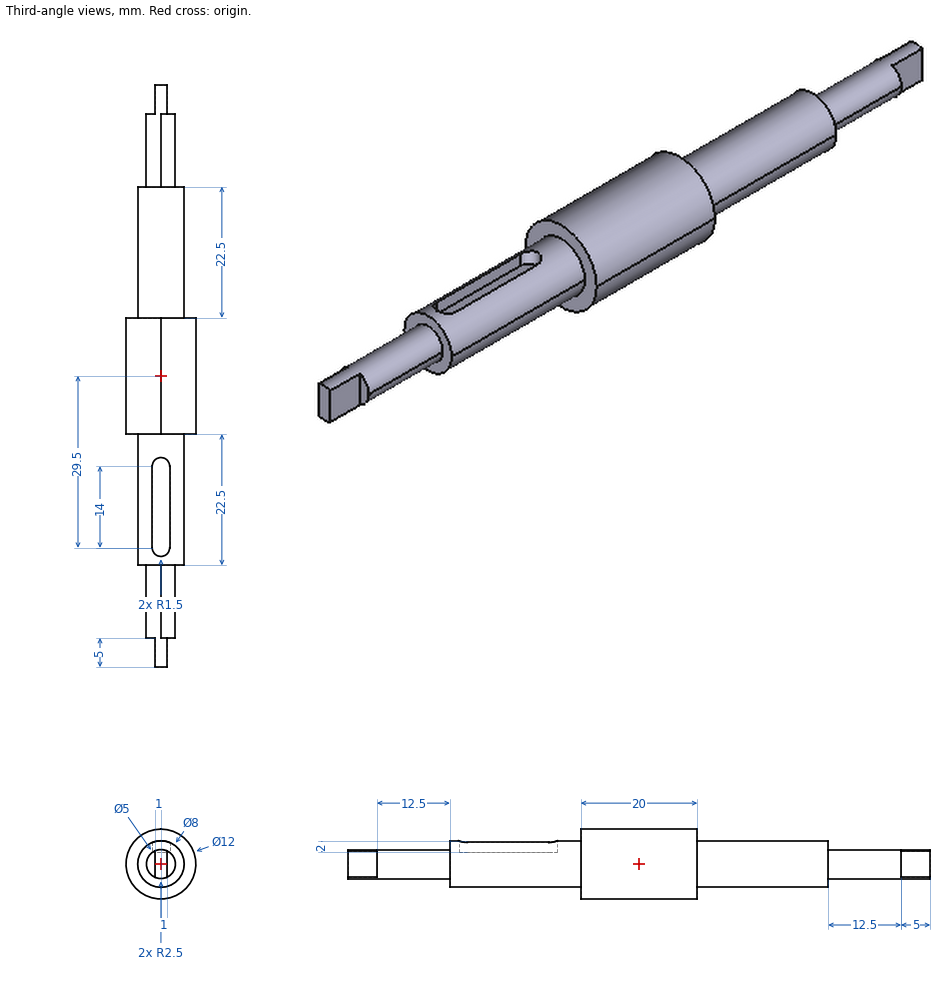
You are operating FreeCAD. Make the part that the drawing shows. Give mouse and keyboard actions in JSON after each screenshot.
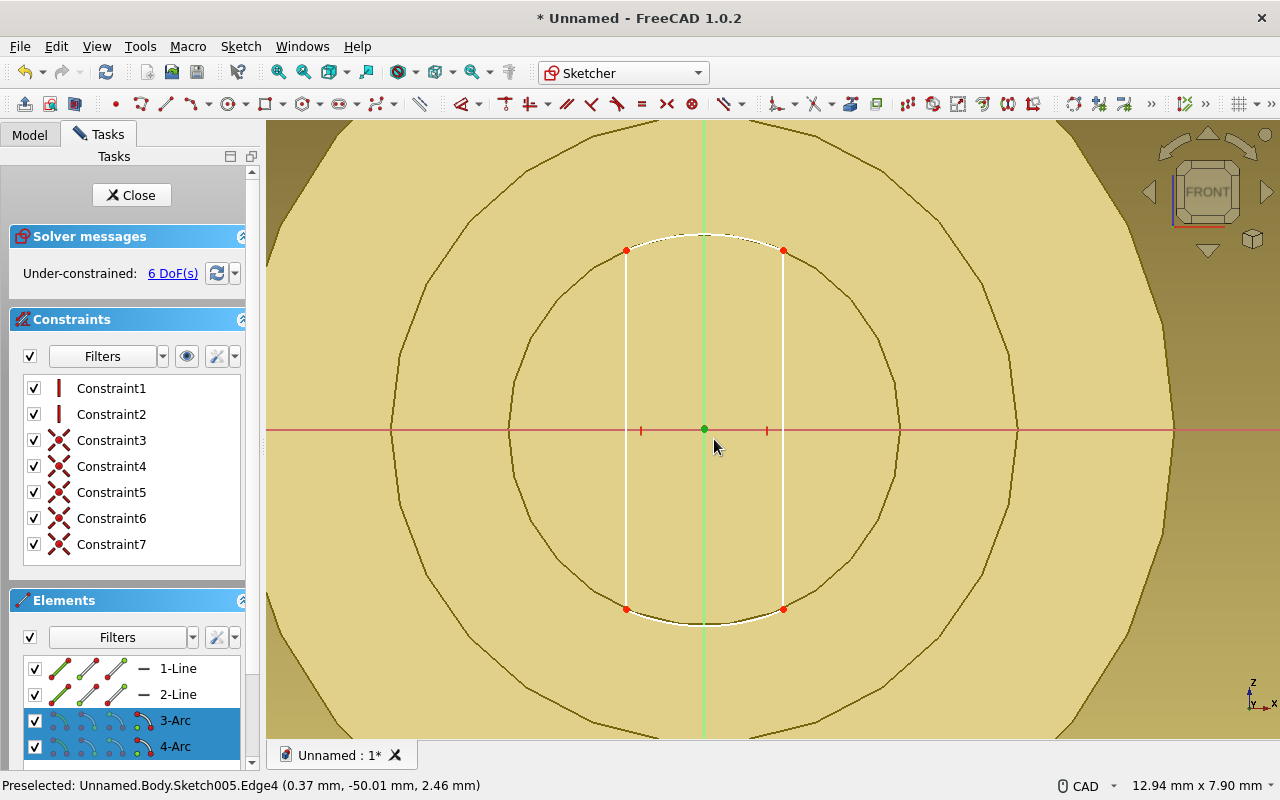
{"action": "left_click", "coordinate": [505, 104]}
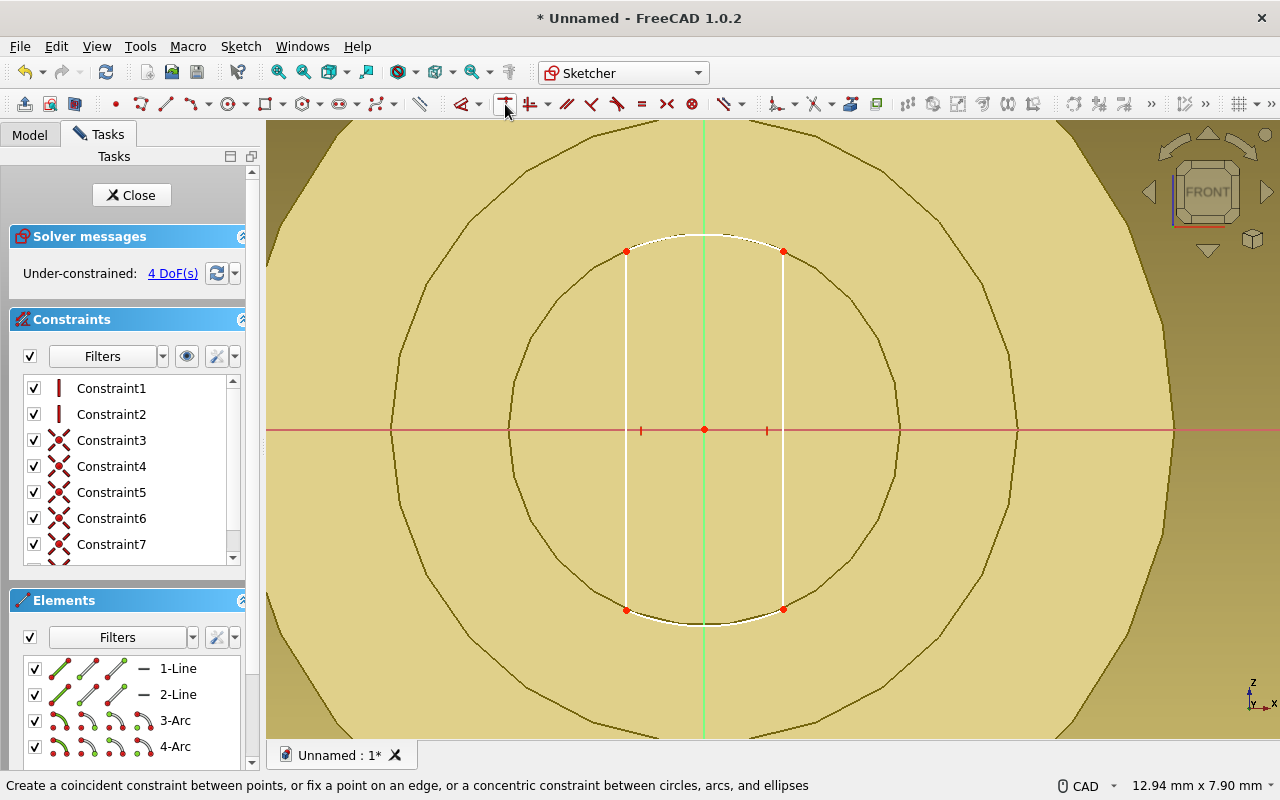
{"action": "left_click", "coordinate": [672, 624]}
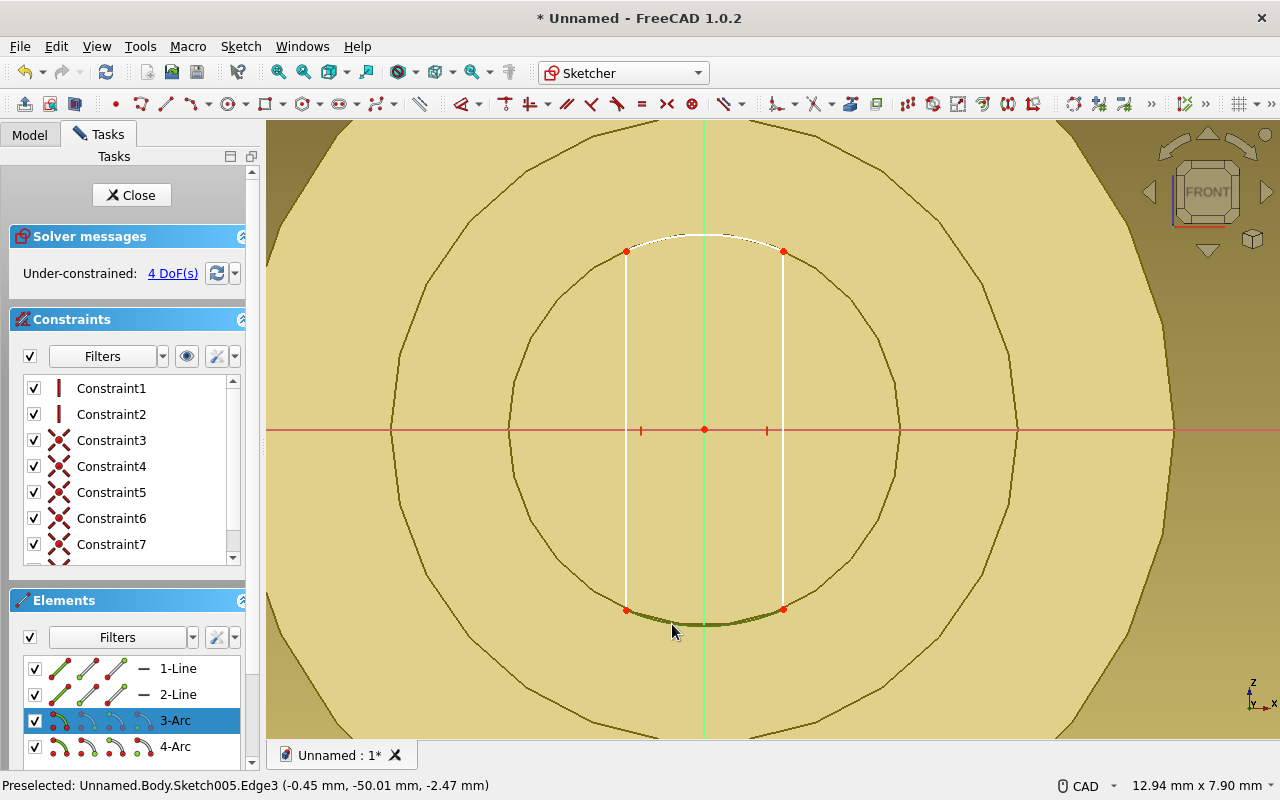
{"action": "left_click", "coordinate": [737, 237]}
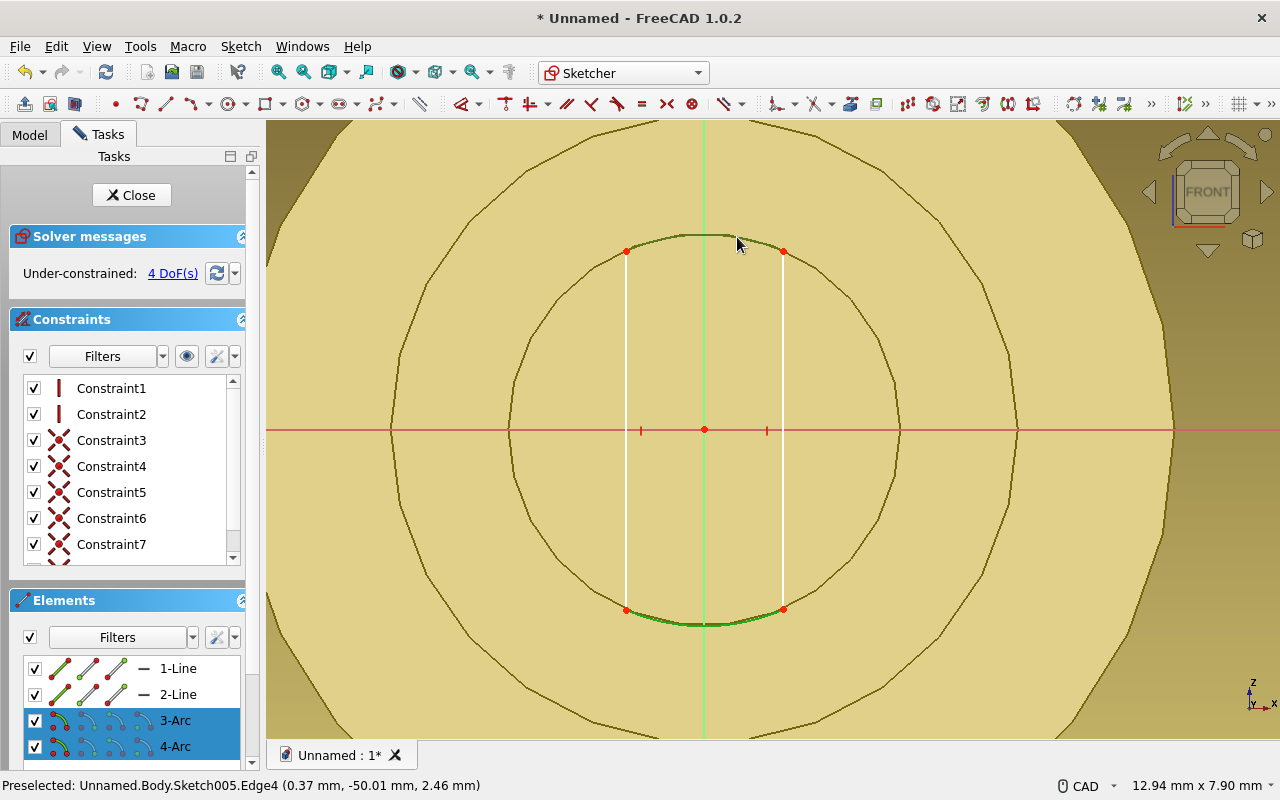
{"action": "key", "text": "e"}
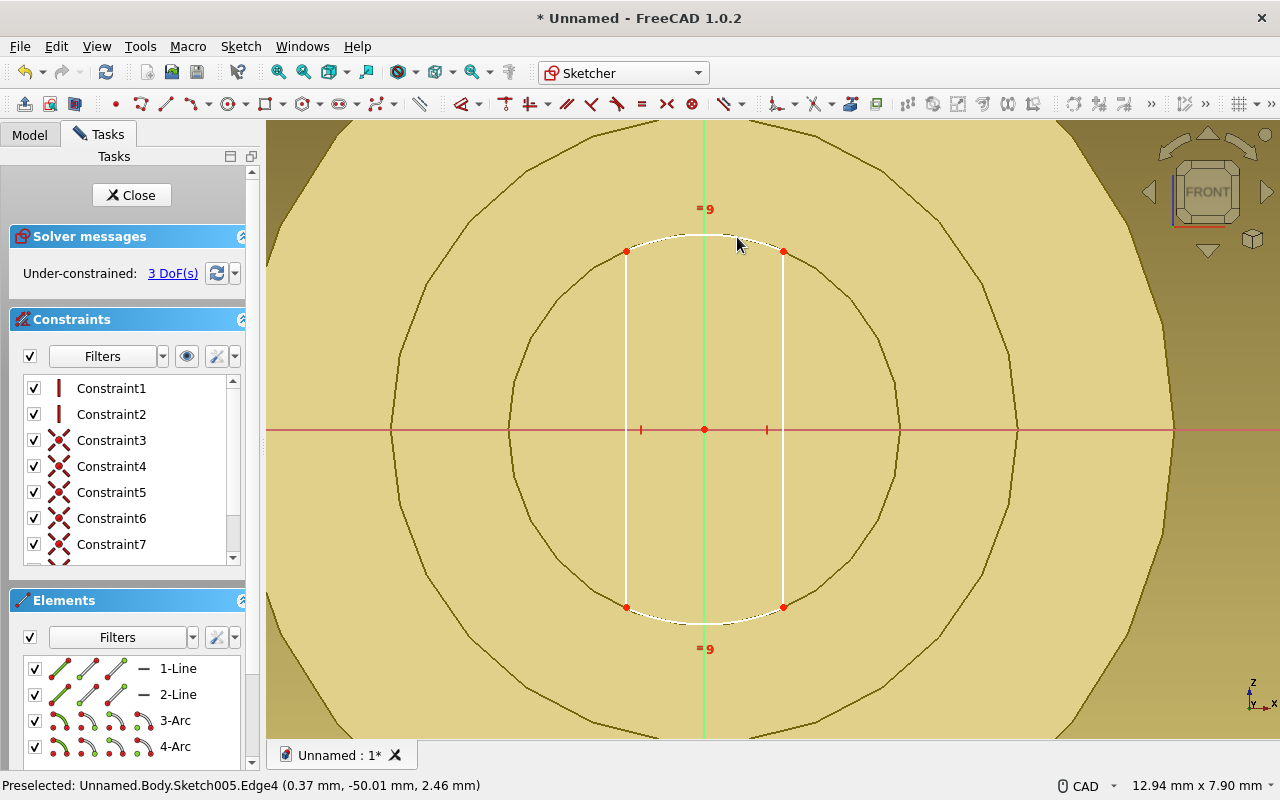
{"action": "key", "text": "d"}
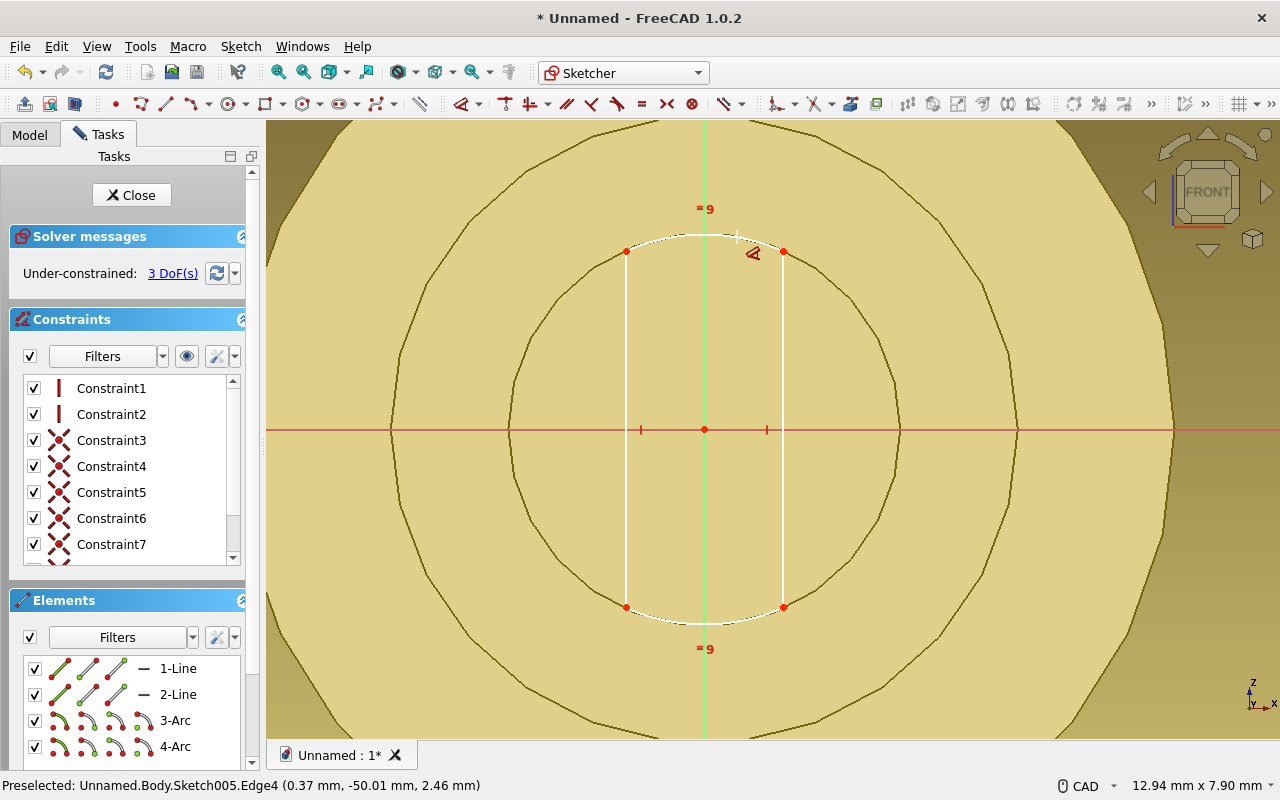
{"action": "left_click", "coordinate": [672, 622]}
{"action": "left_click", "coordinate": [667, 654]}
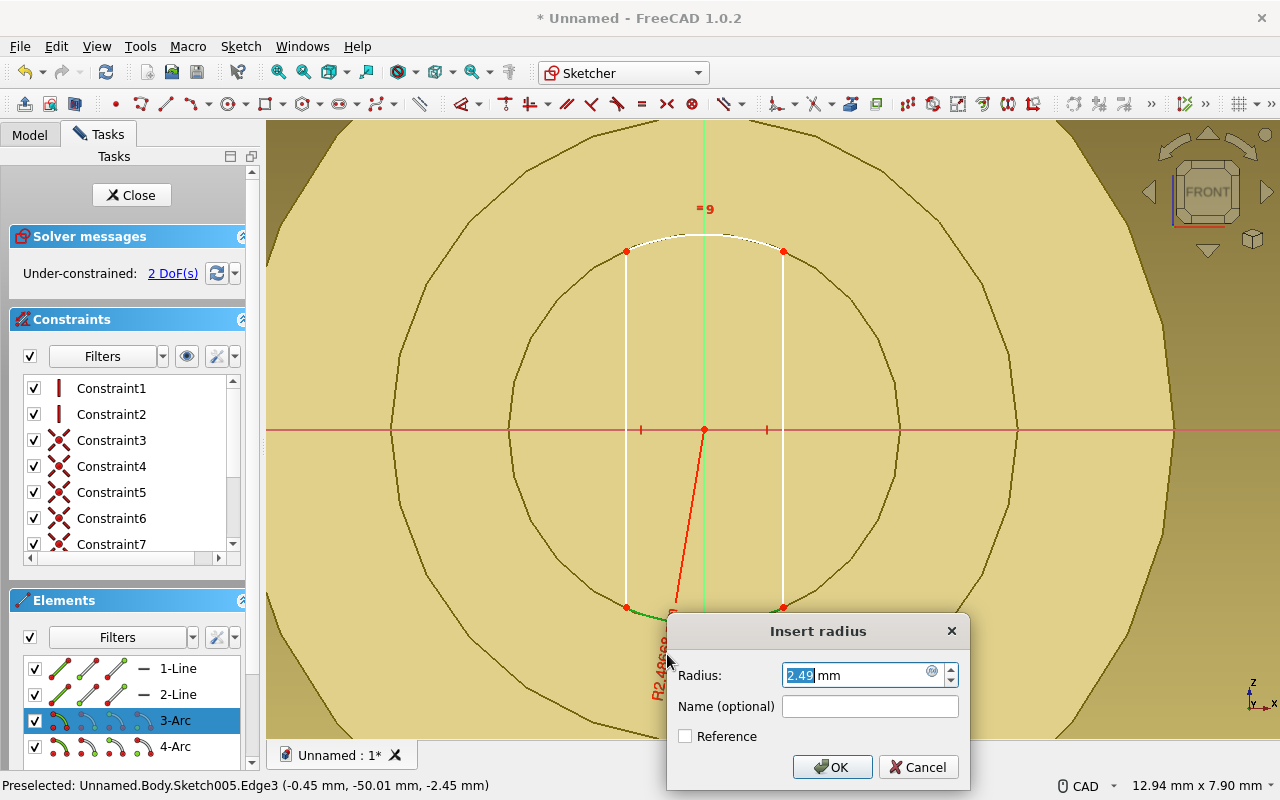
{"action": "type", "text": "2.5"}
{"action": "key", "text": "Return"}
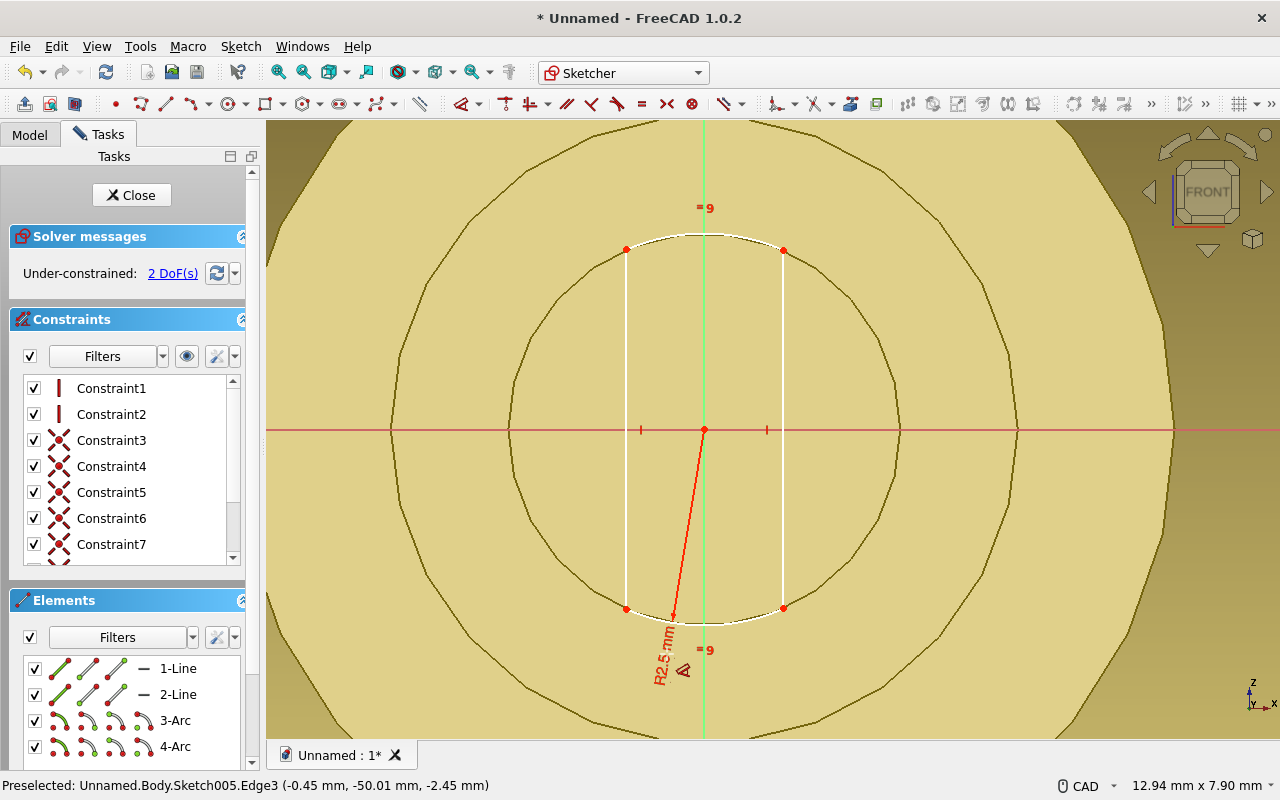
{"action": "left_click", "coordinate": [626, 250]}
{"action": "left_click", "coordinate": [665, 216]}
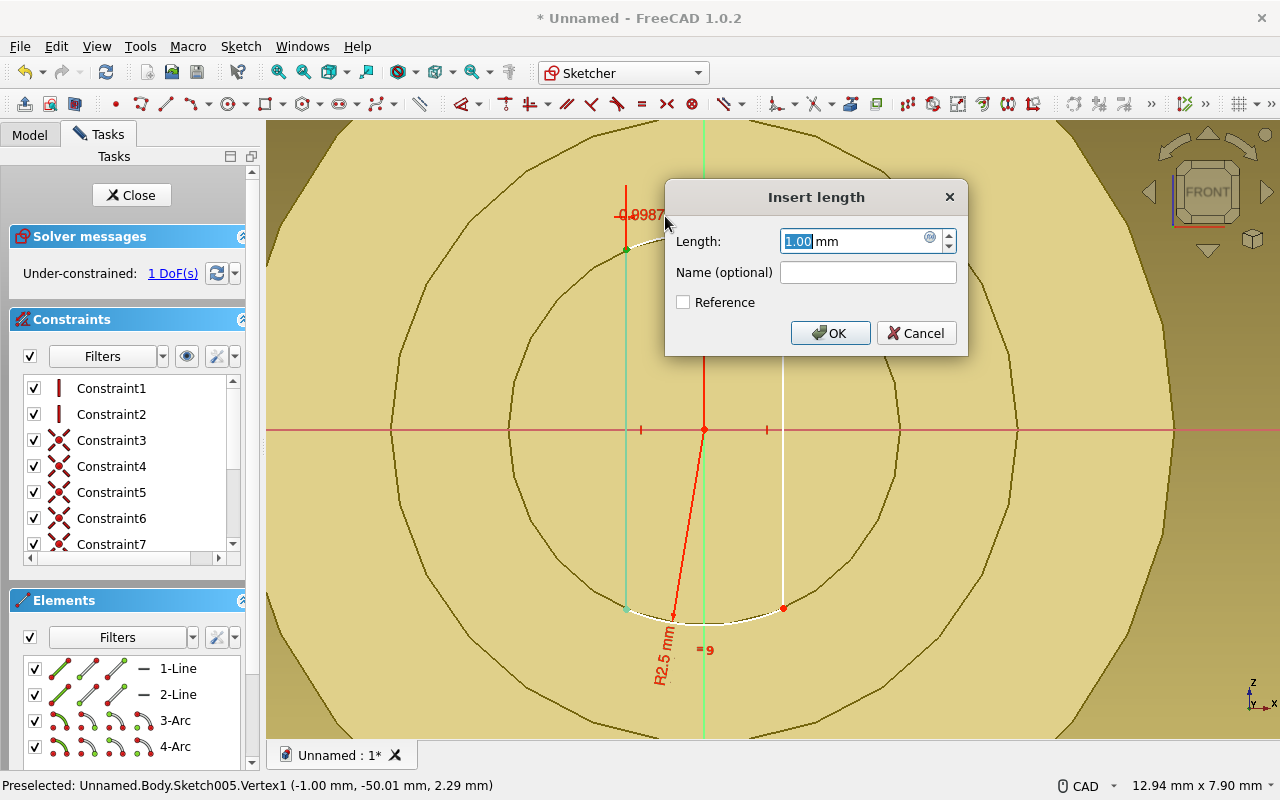
{"action": "type", "text": "1"}
{"action": "key", "text": "Return"}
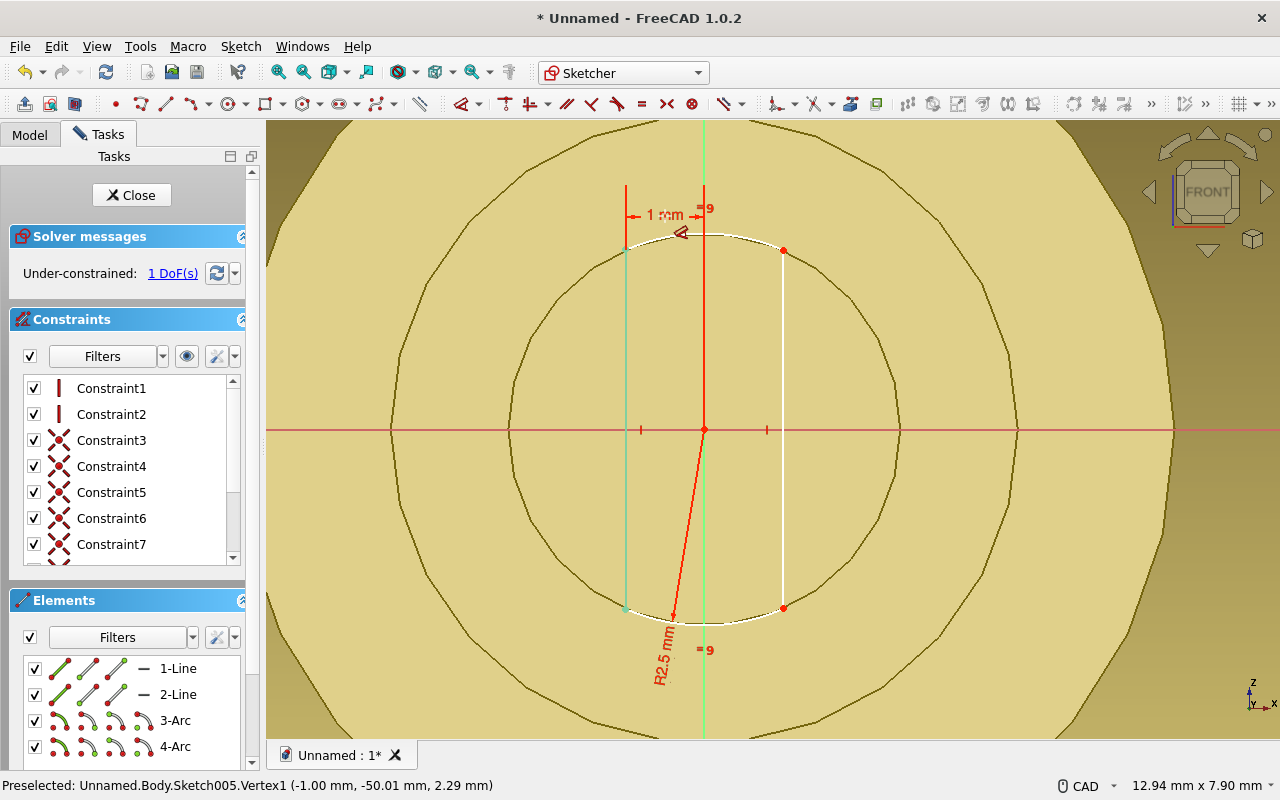
{"action": "left_click", "coordinate": [783, 609]}
{"action": "left_click", "coordinate": [744, 643]}